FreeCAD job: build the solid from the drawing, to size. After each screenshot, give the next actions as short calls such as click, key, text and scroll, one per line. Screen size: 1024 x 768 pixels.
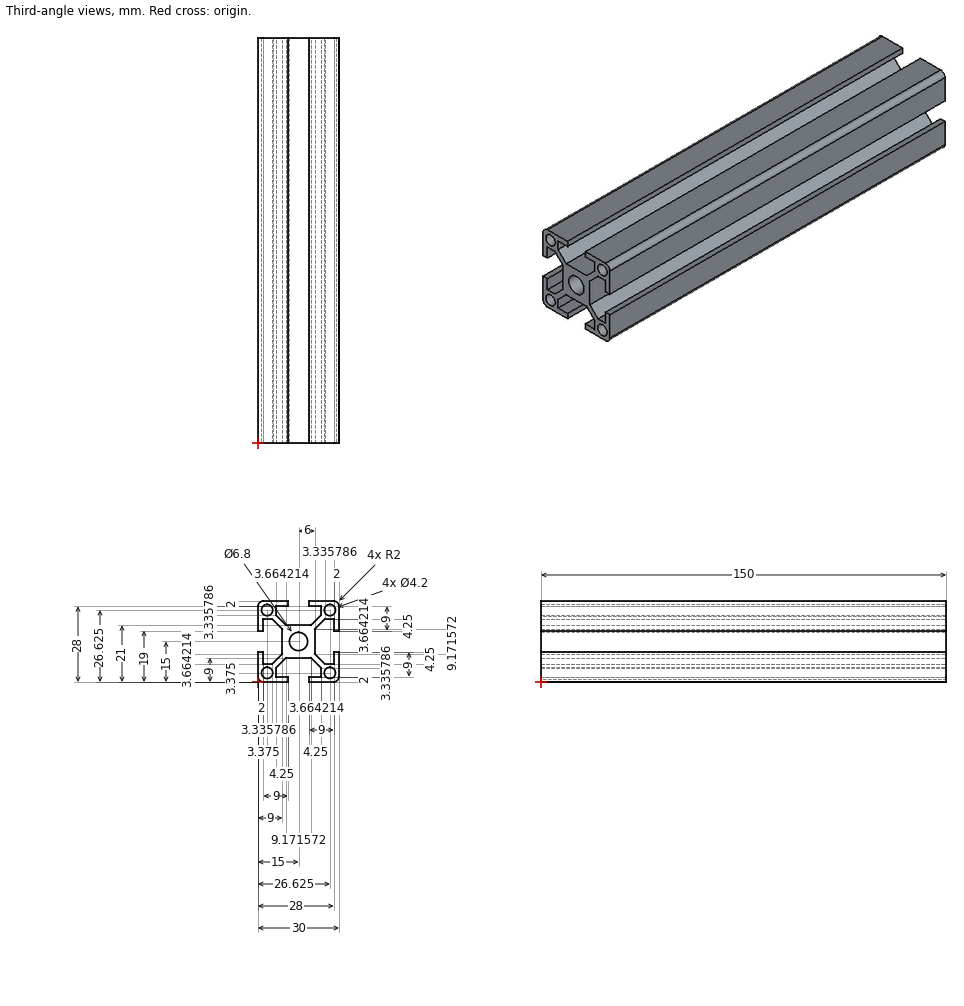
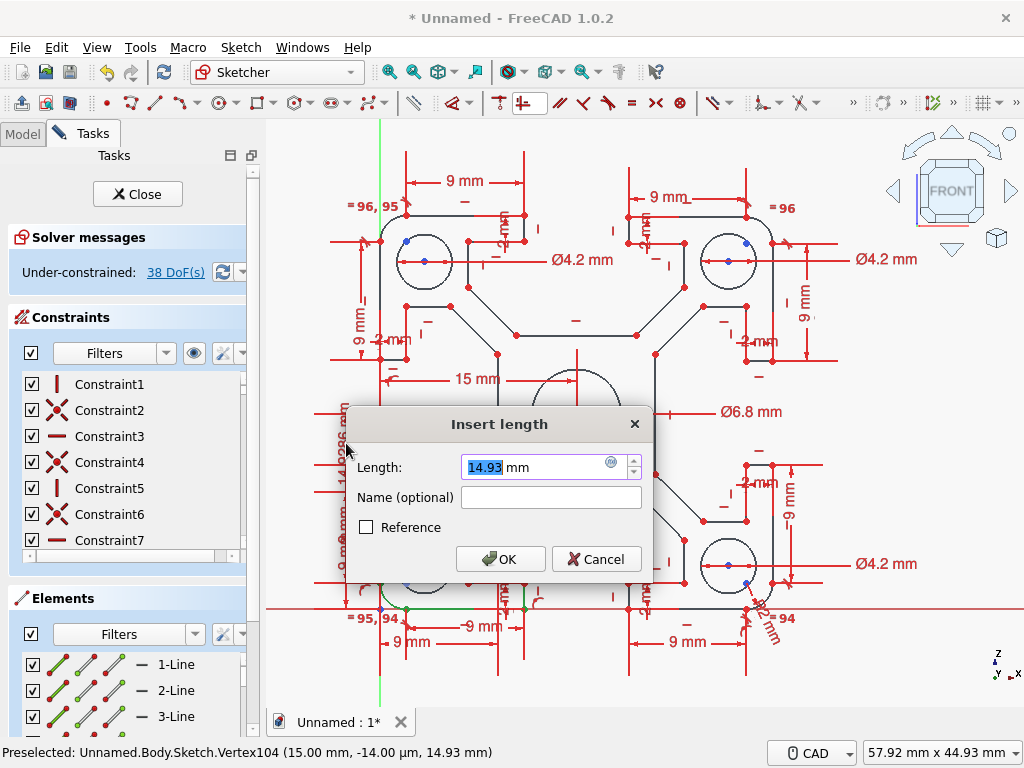
text(15)
key(Return)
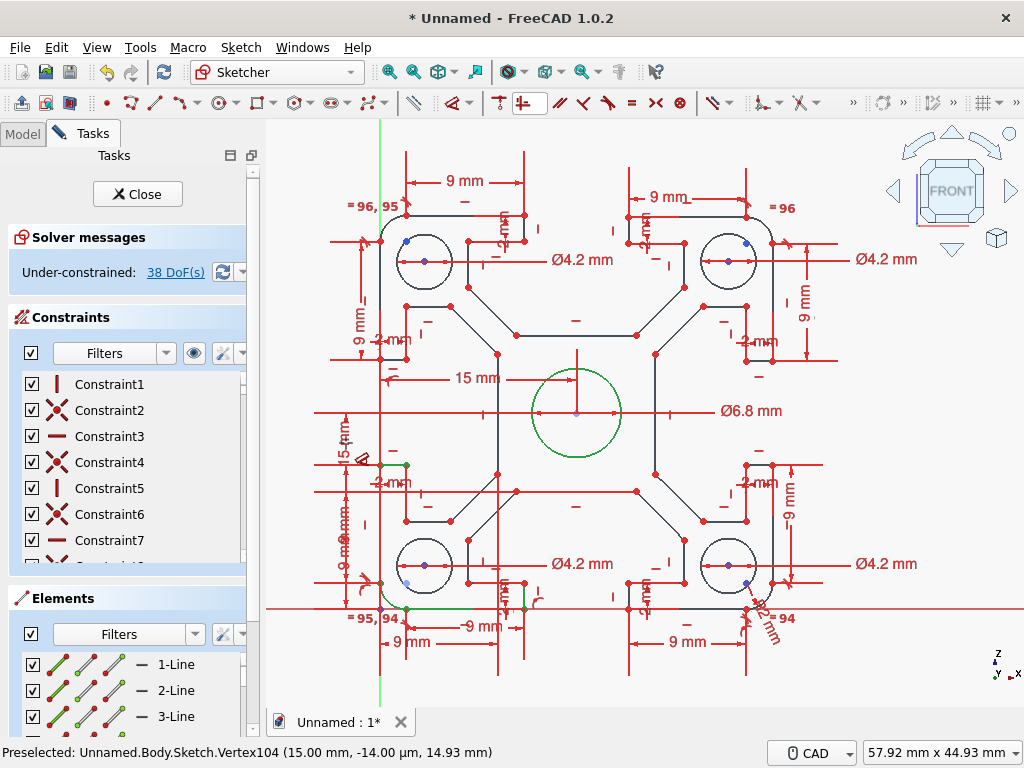
click(655, 355)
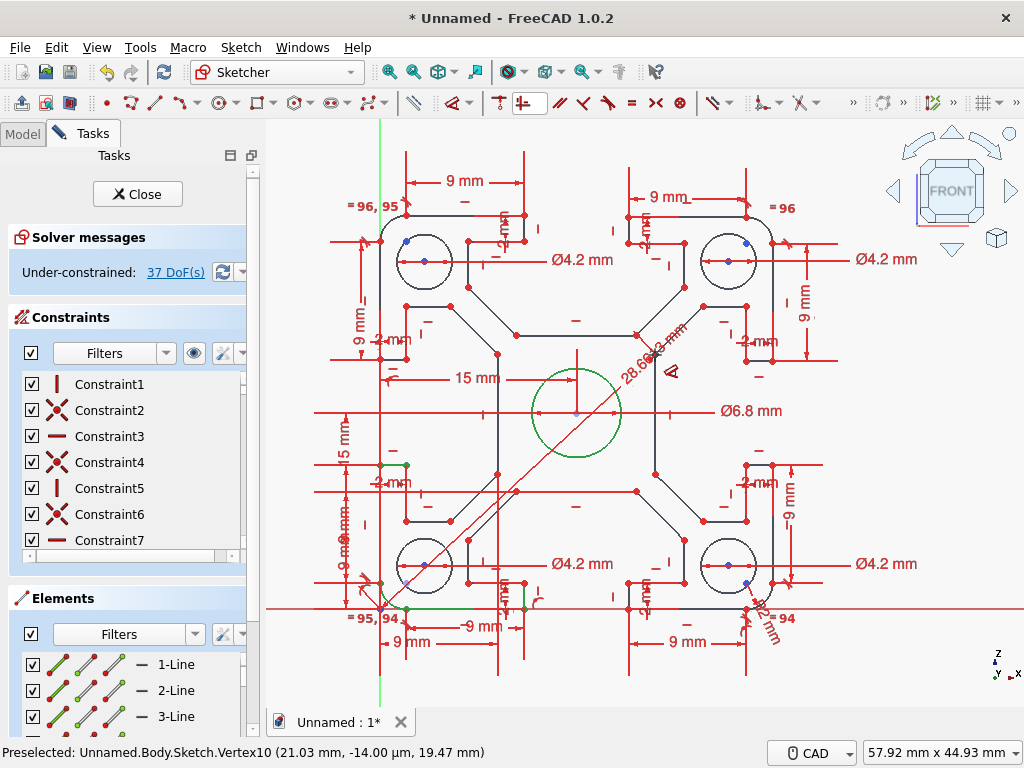
click(577, 413)
click(616, 321)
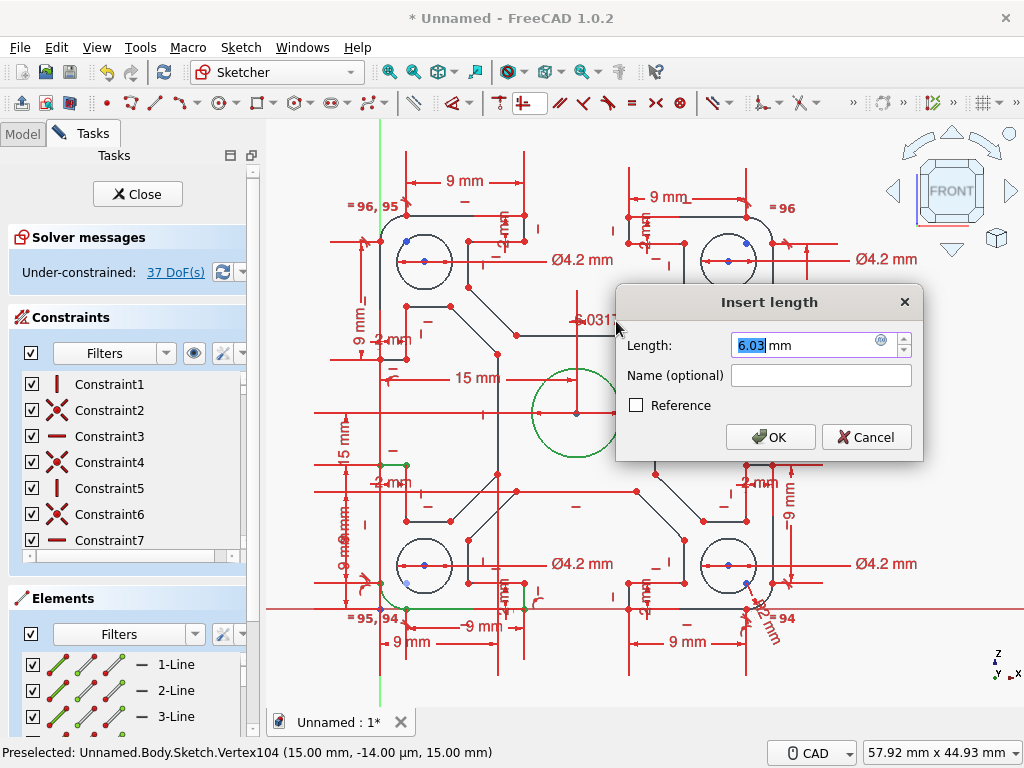
text(6)
key(Return)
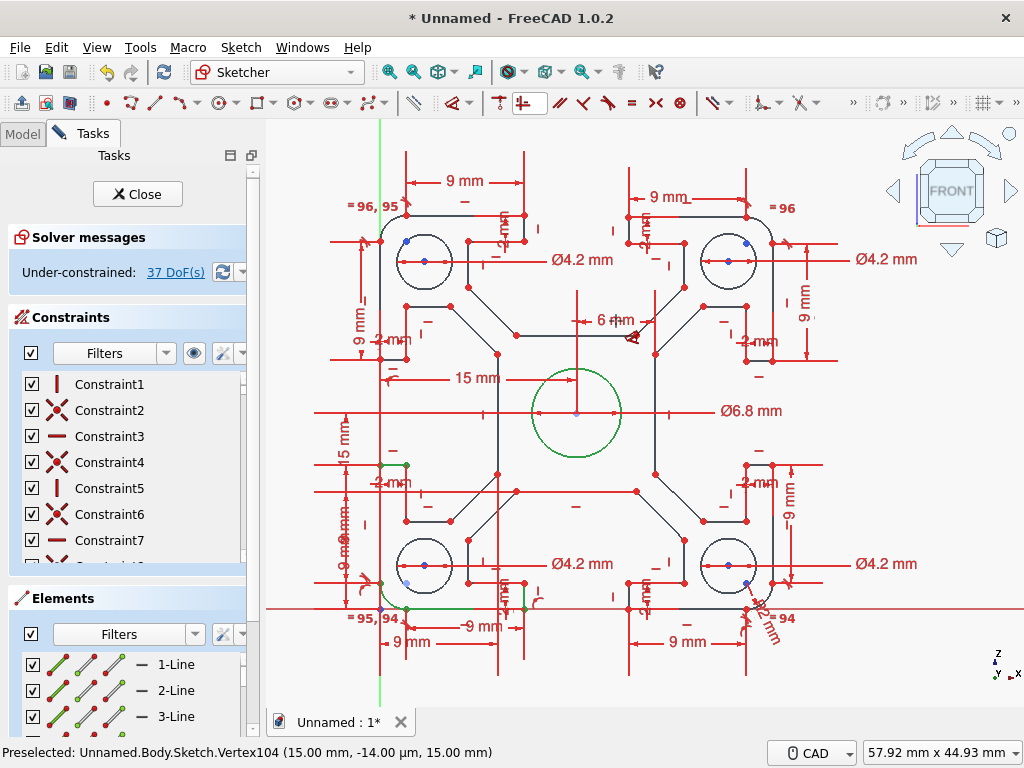
click(773, 244)
click(576, 643)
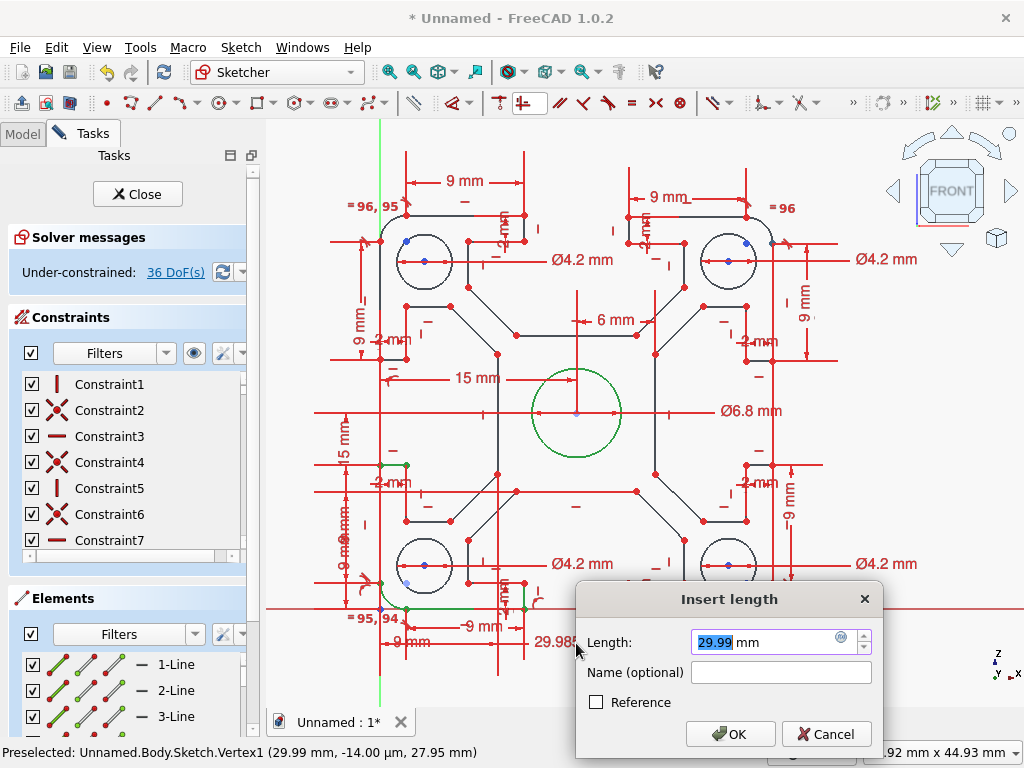
text(30)
key(Return)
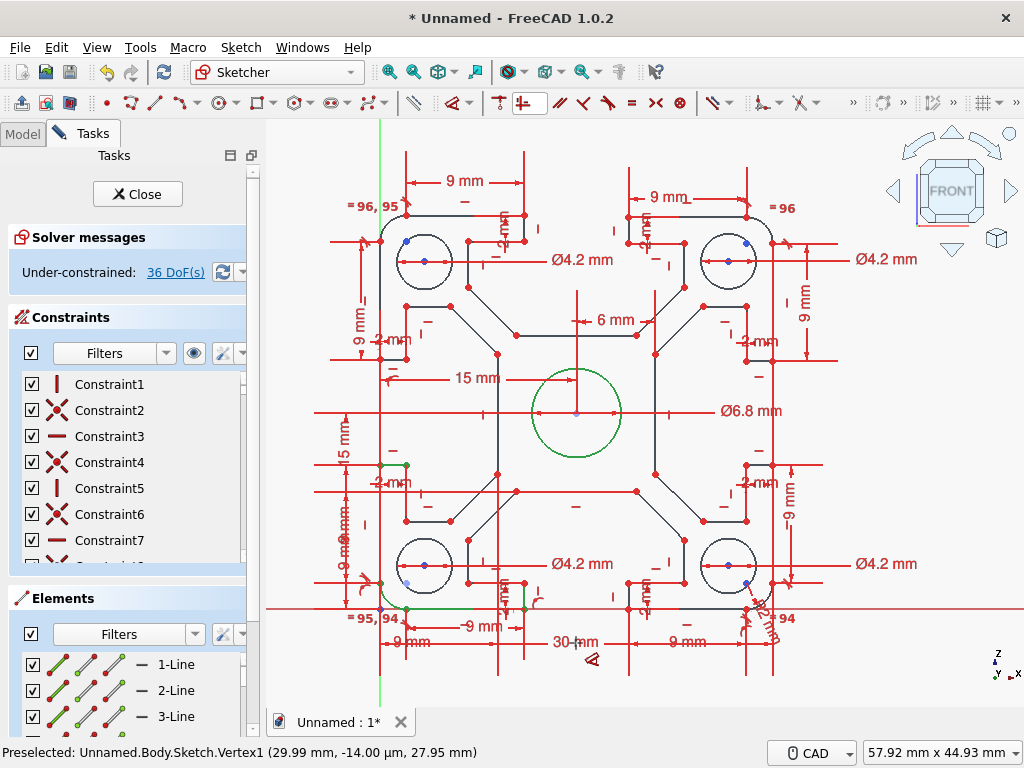
click(773, 244)
click(346, 298)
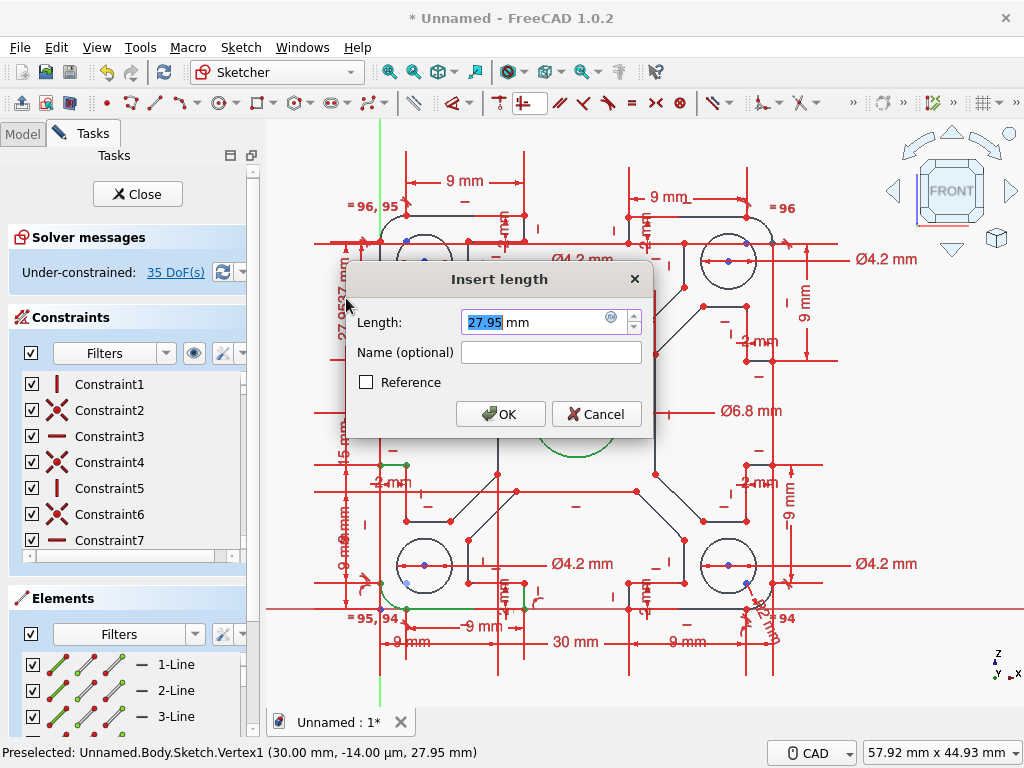
text(28)
key(Return)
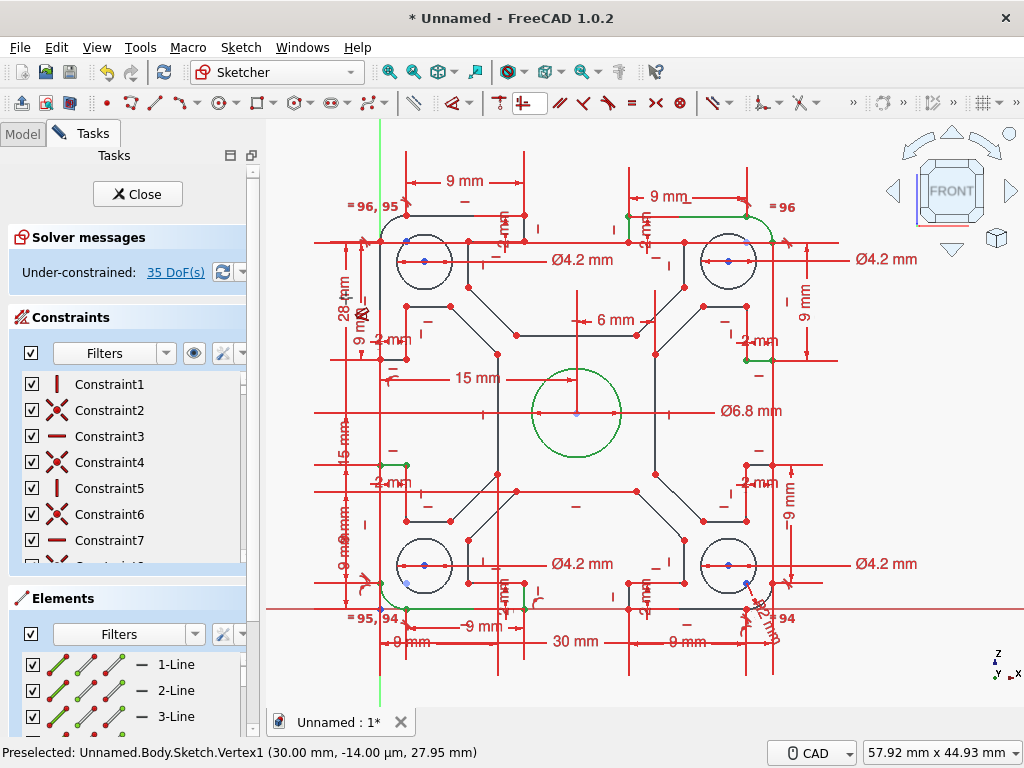
click(746, 522)
click(563, 667)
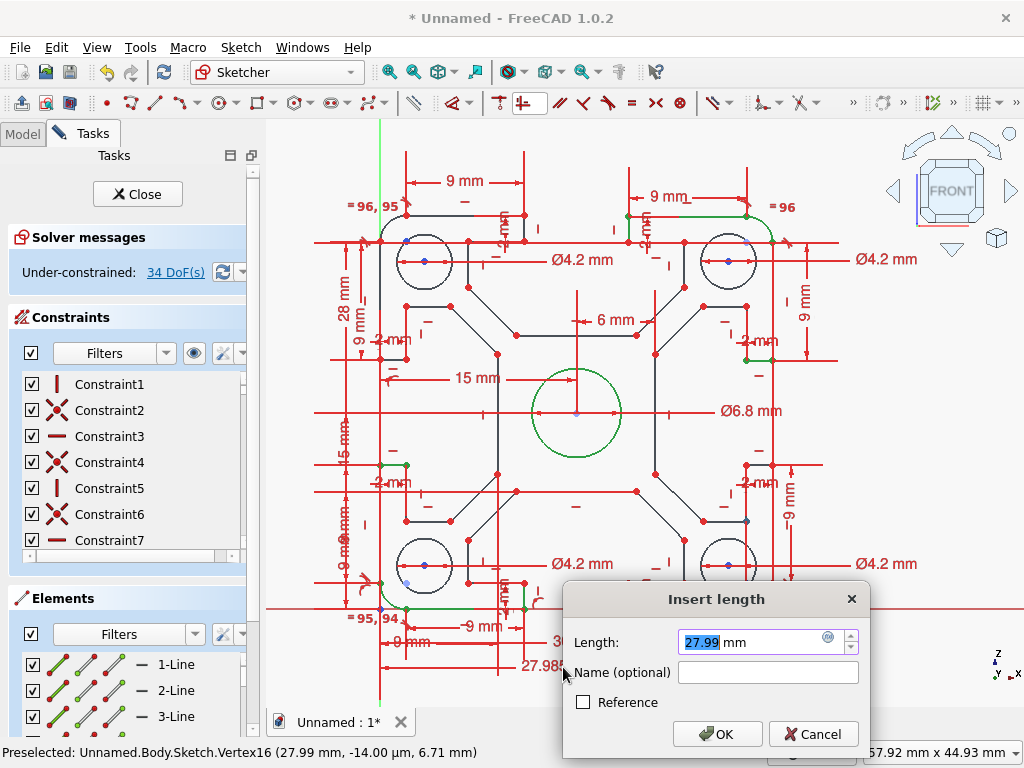
text(28)
key(Return)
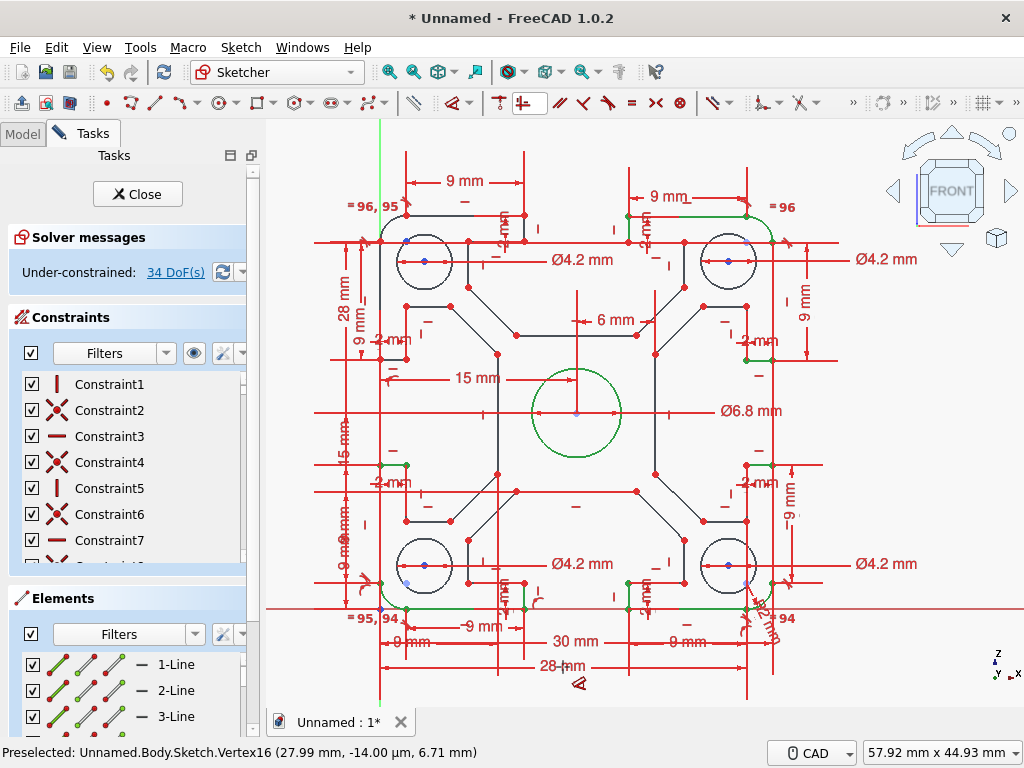
click(406, 360)
click(346, 397)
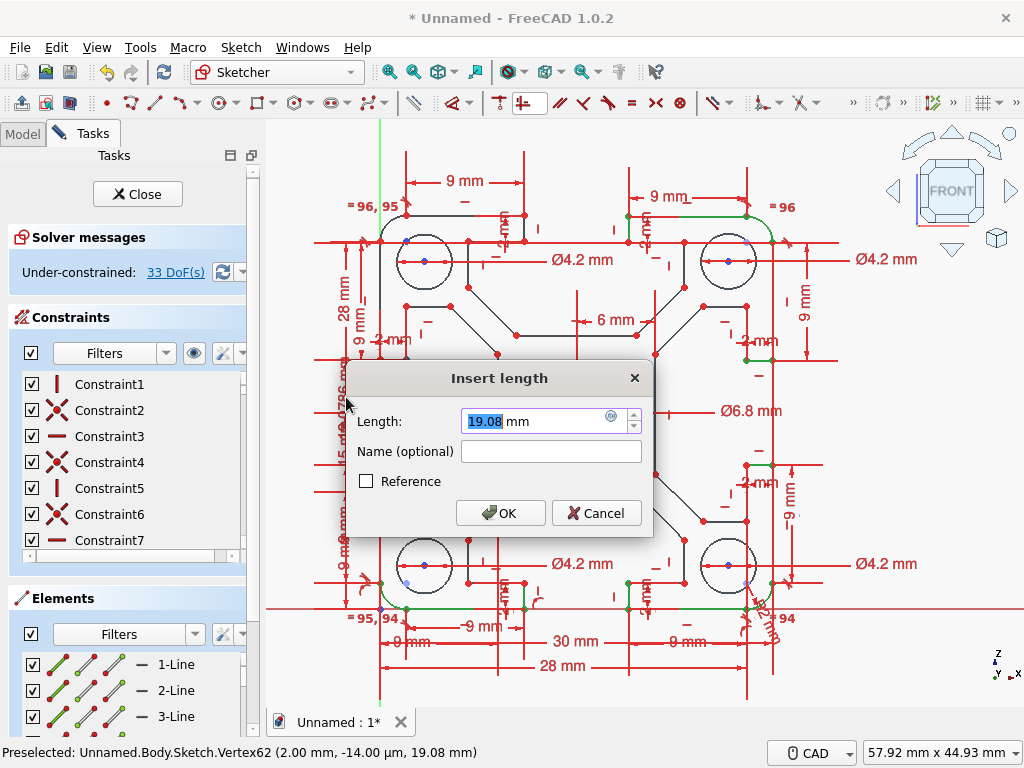
text(19)
key(Return)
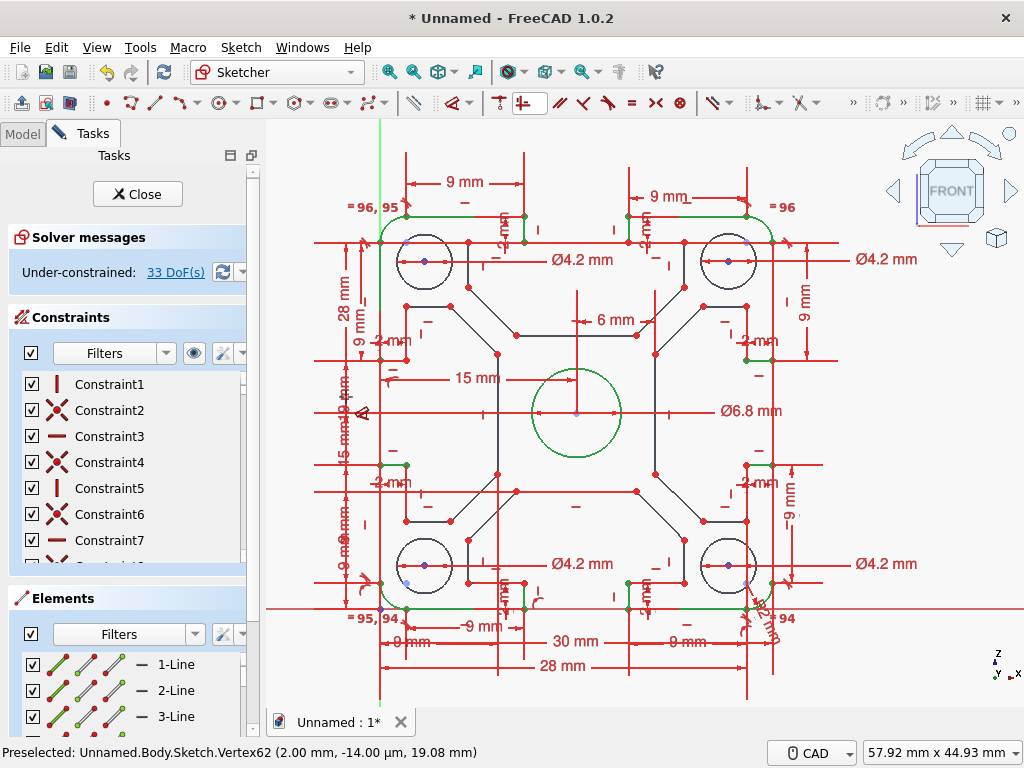
click(516, 336)
click(346, 377)